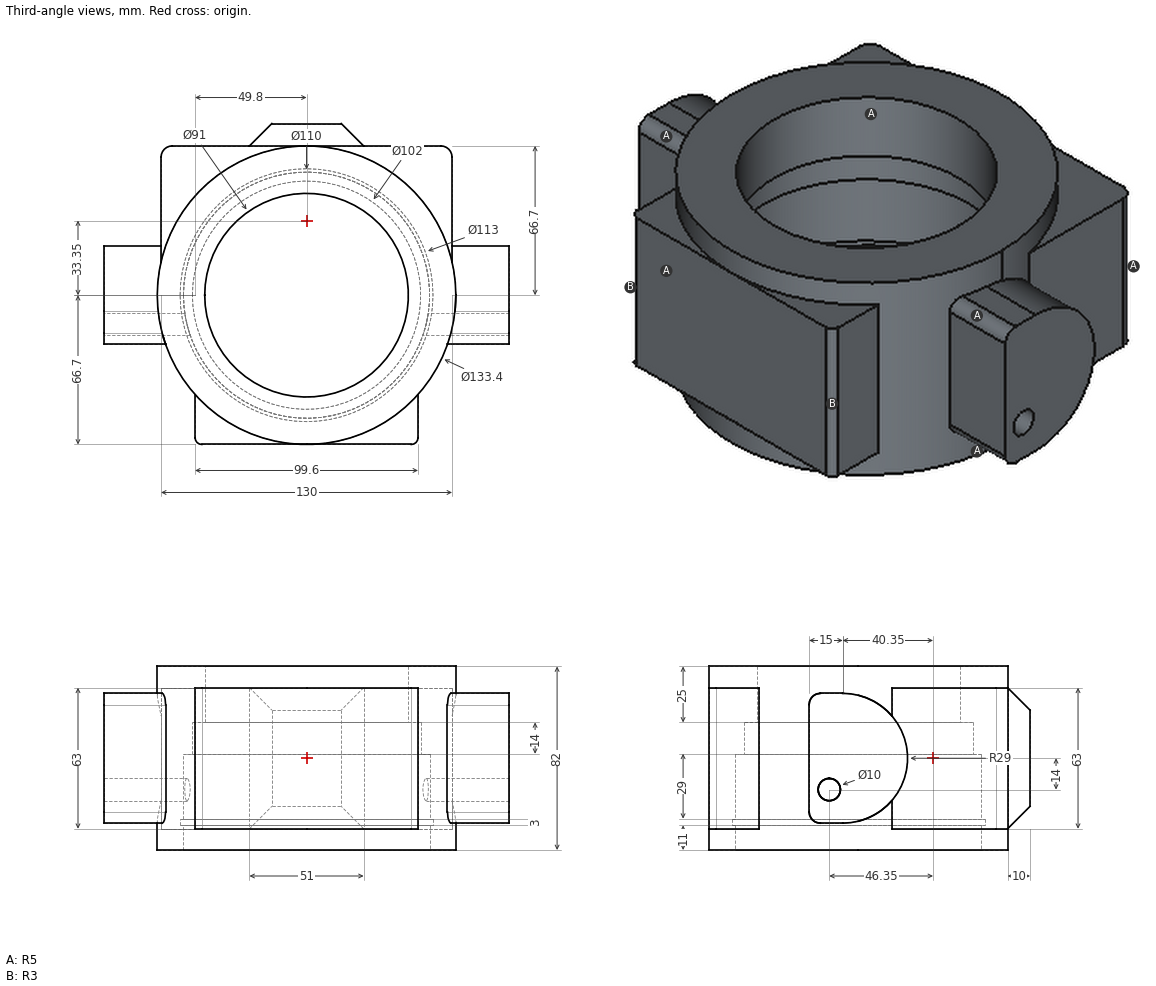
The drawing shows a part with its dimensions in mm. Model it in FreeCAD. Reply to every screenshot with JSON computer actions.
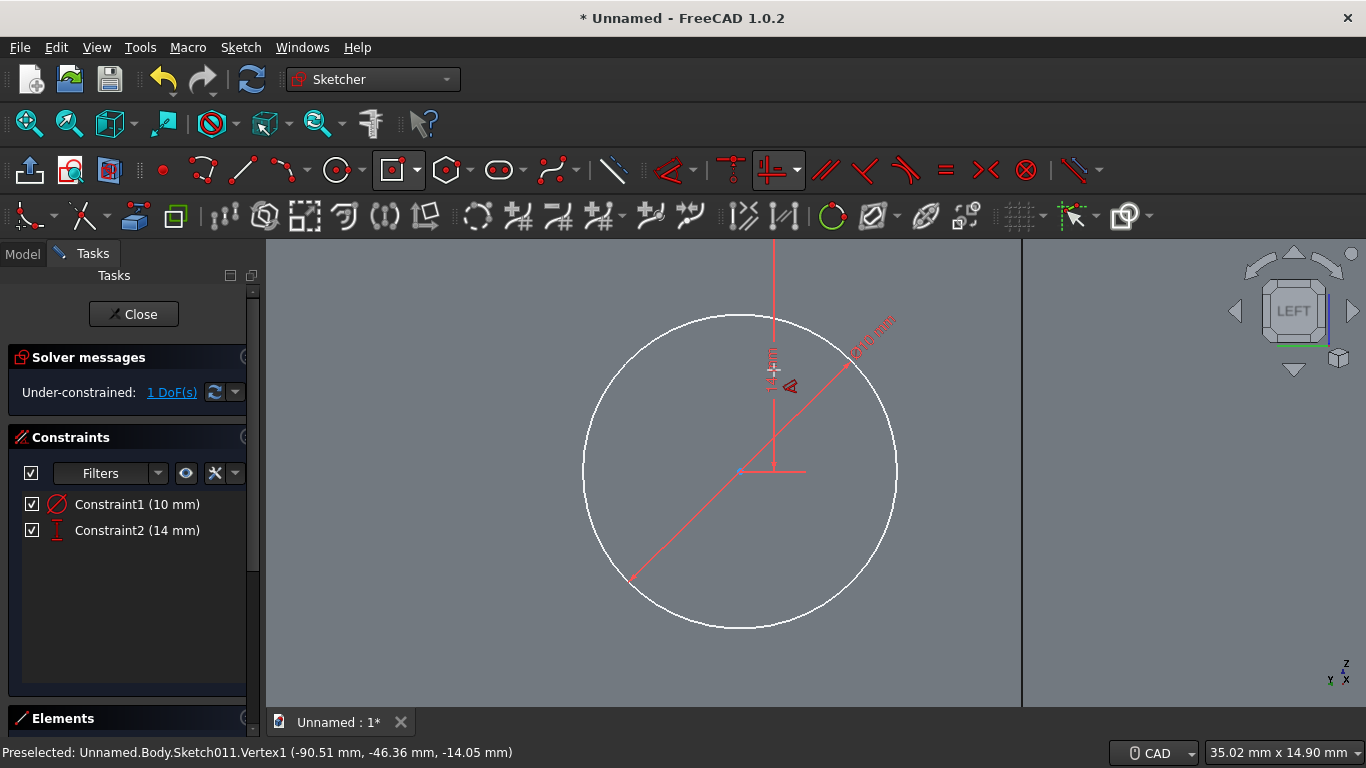
{"action": "left_click", "coordinate": [740, 472]}
{"action": "left_click", "coordinate": [517, 506]}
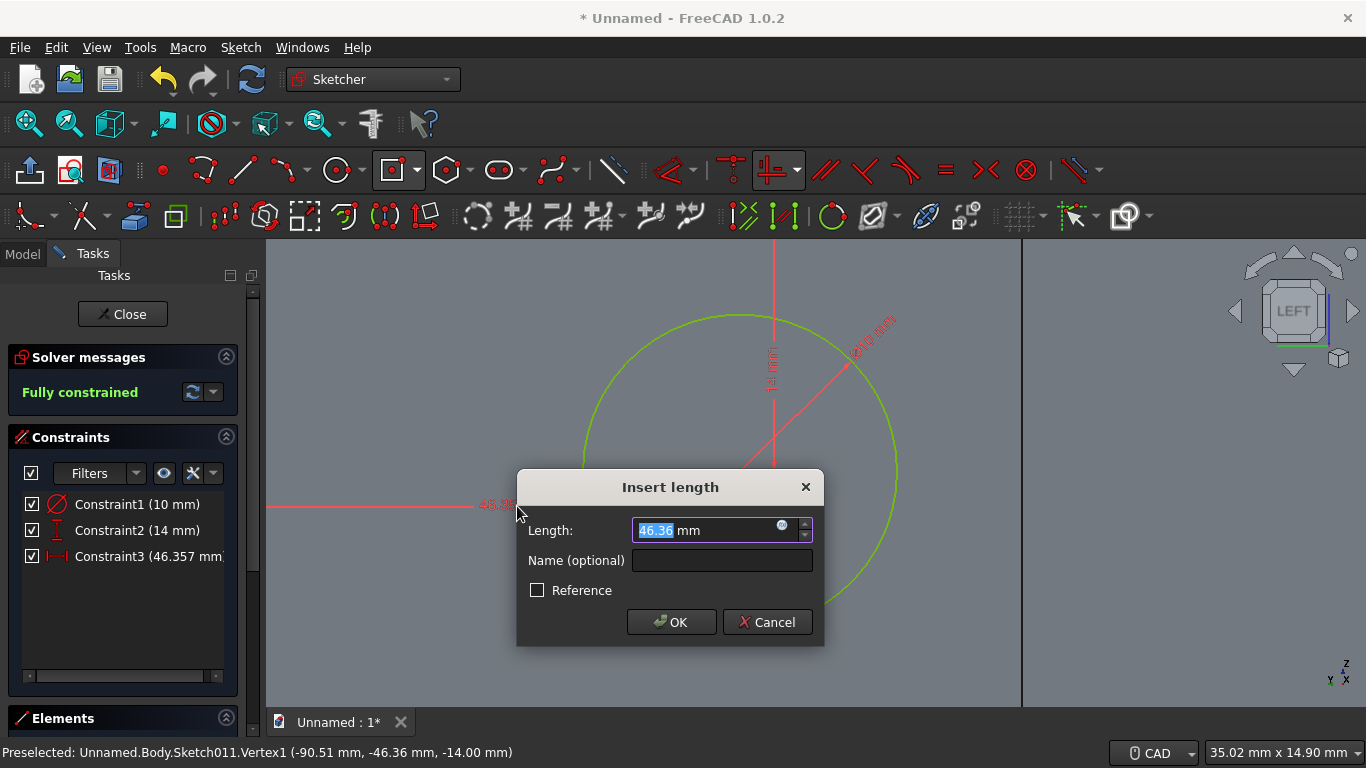
{"action": "type", "text": "46.35"}
{"action": "key", "text": "Return"}
{"action": "key", "text": "Escape"}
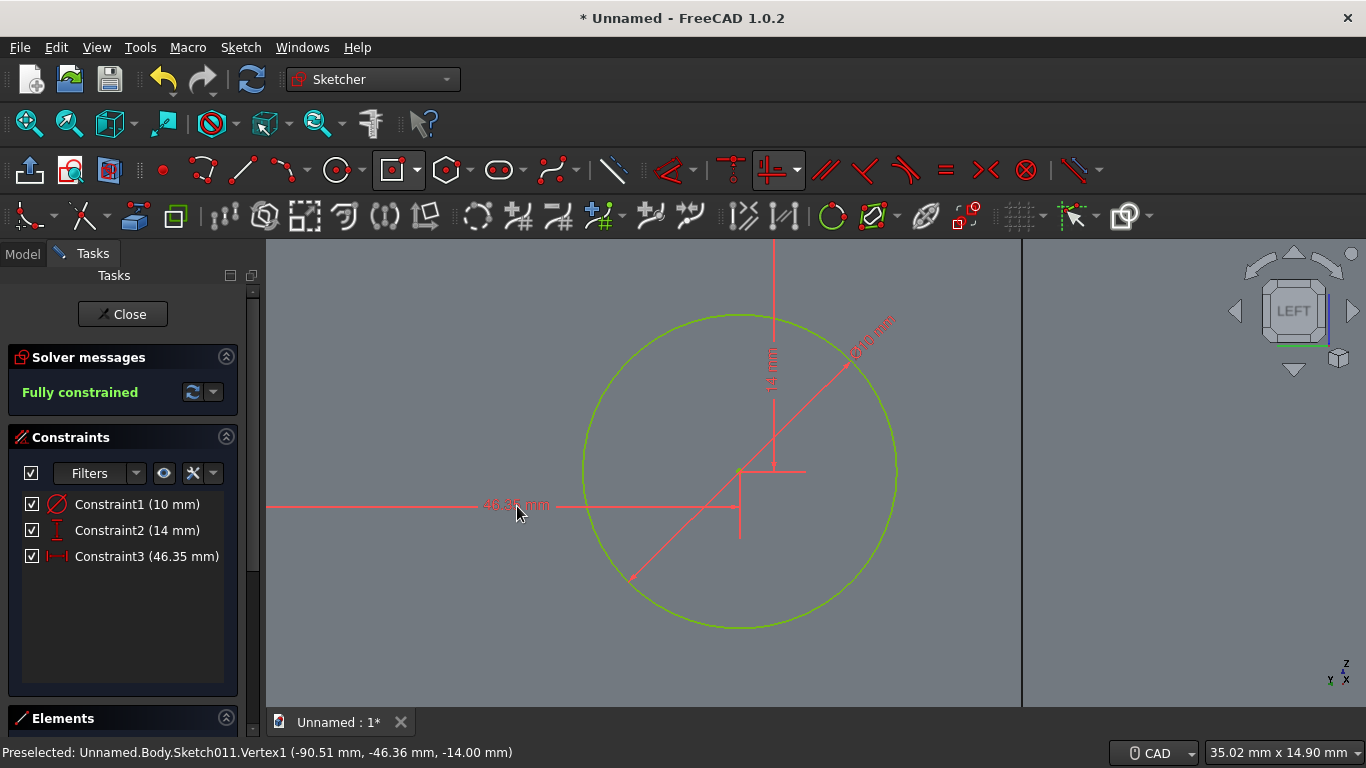
{"action": "left_click", "coordinate": [123, 314]}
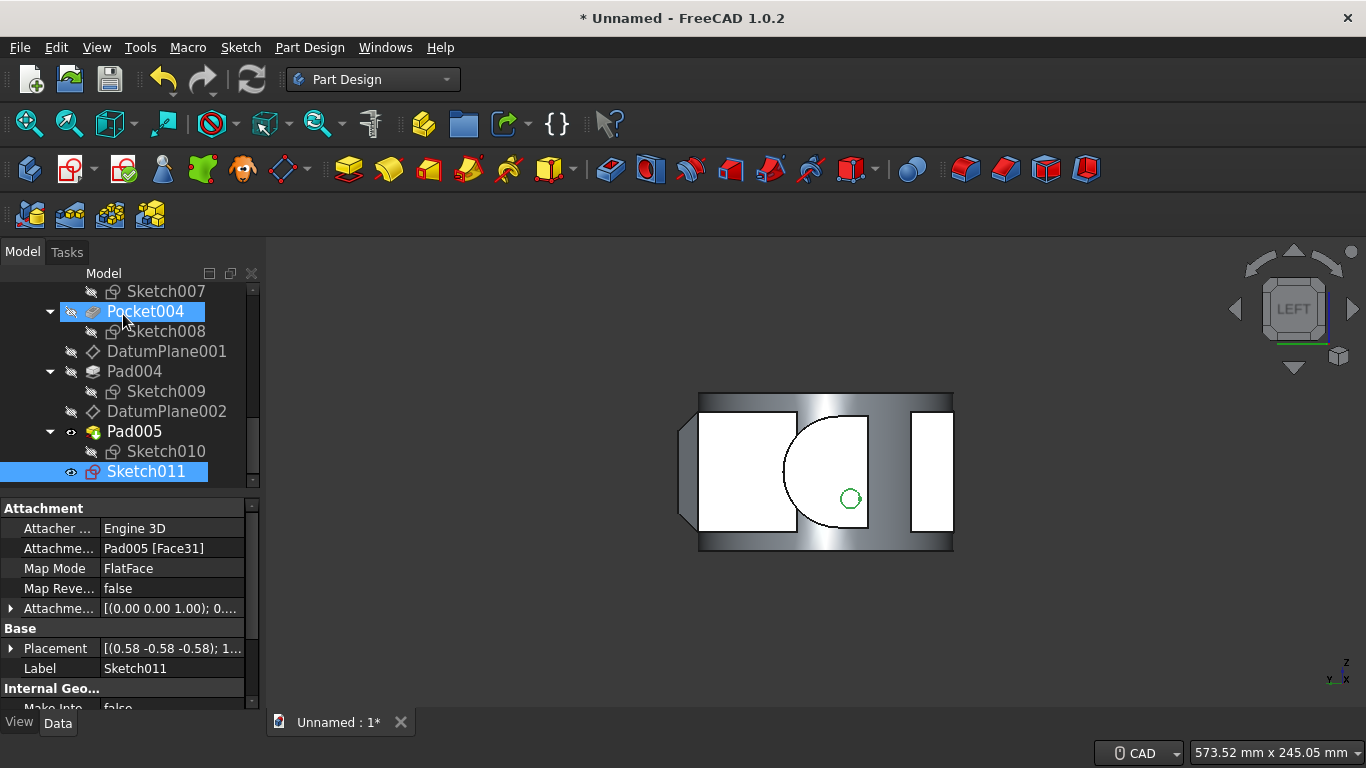
{"action": "left_click", "coordinate": [612, 170]}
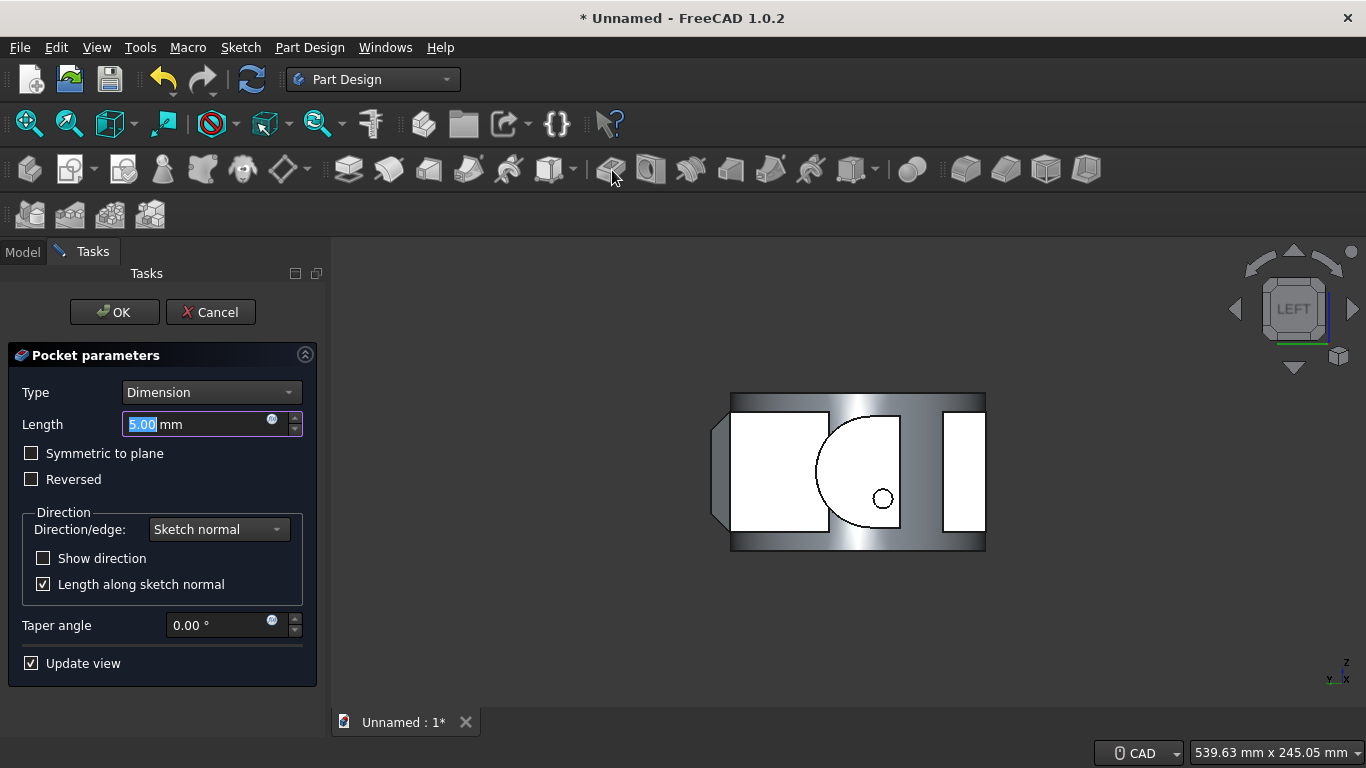
{"action": "left_click", "coordinate": [212, 392]}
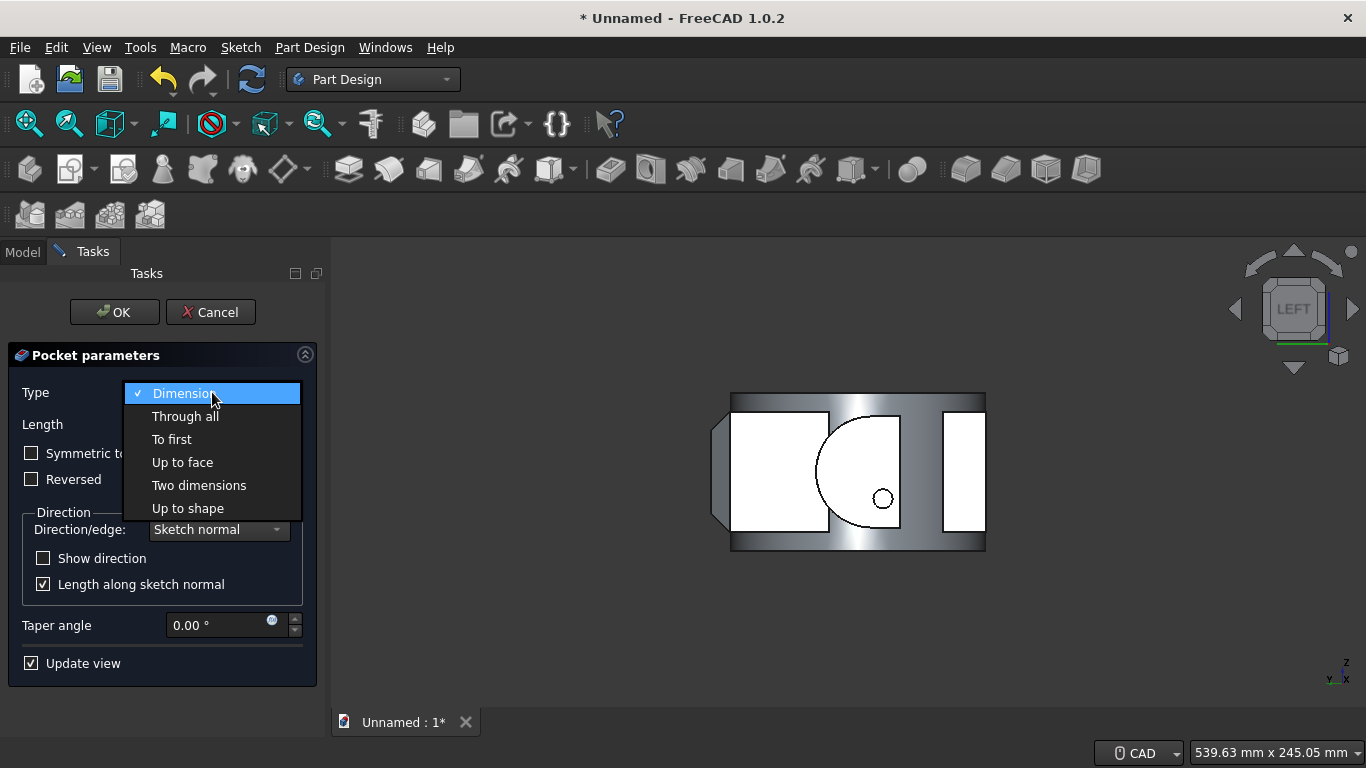
{"action": "left_click", "coordinate": [212, 416]}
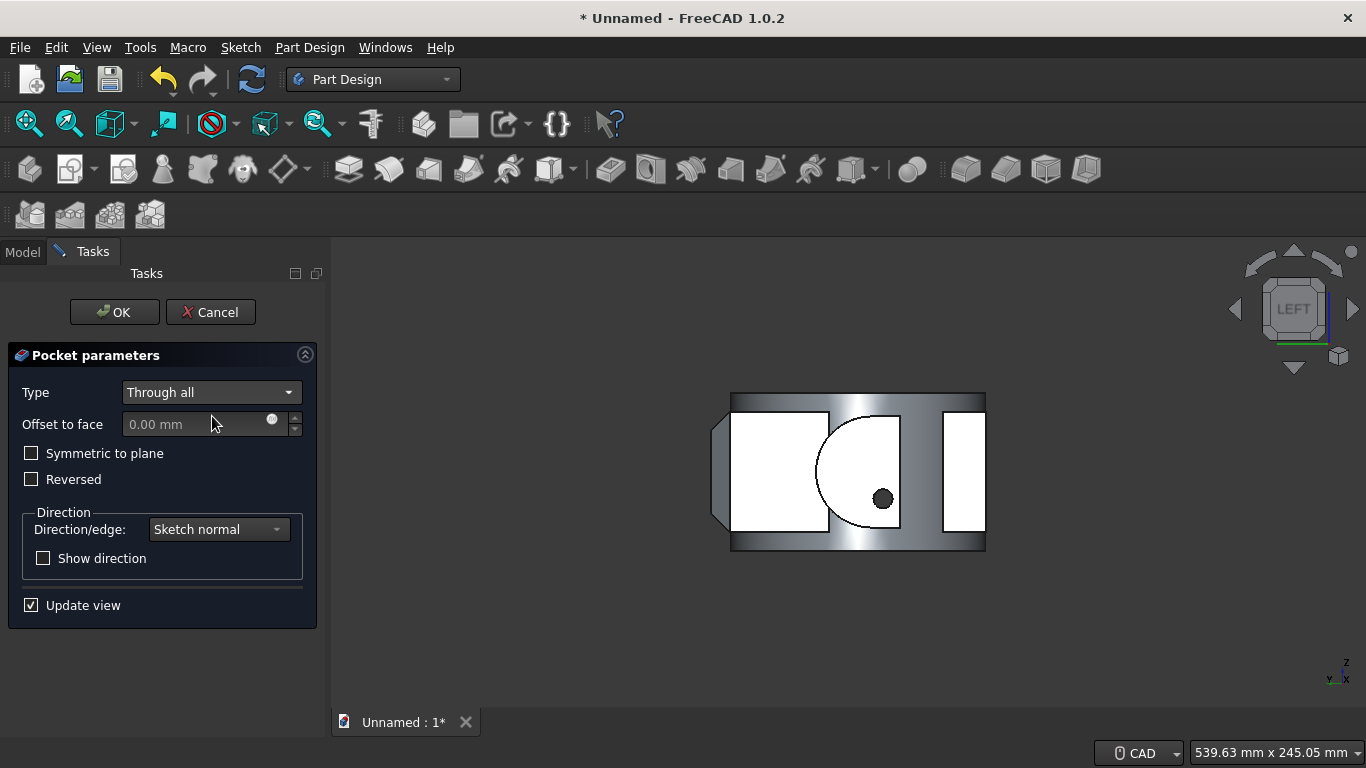
{"action": "left_click", "coordinate": [115, 312]}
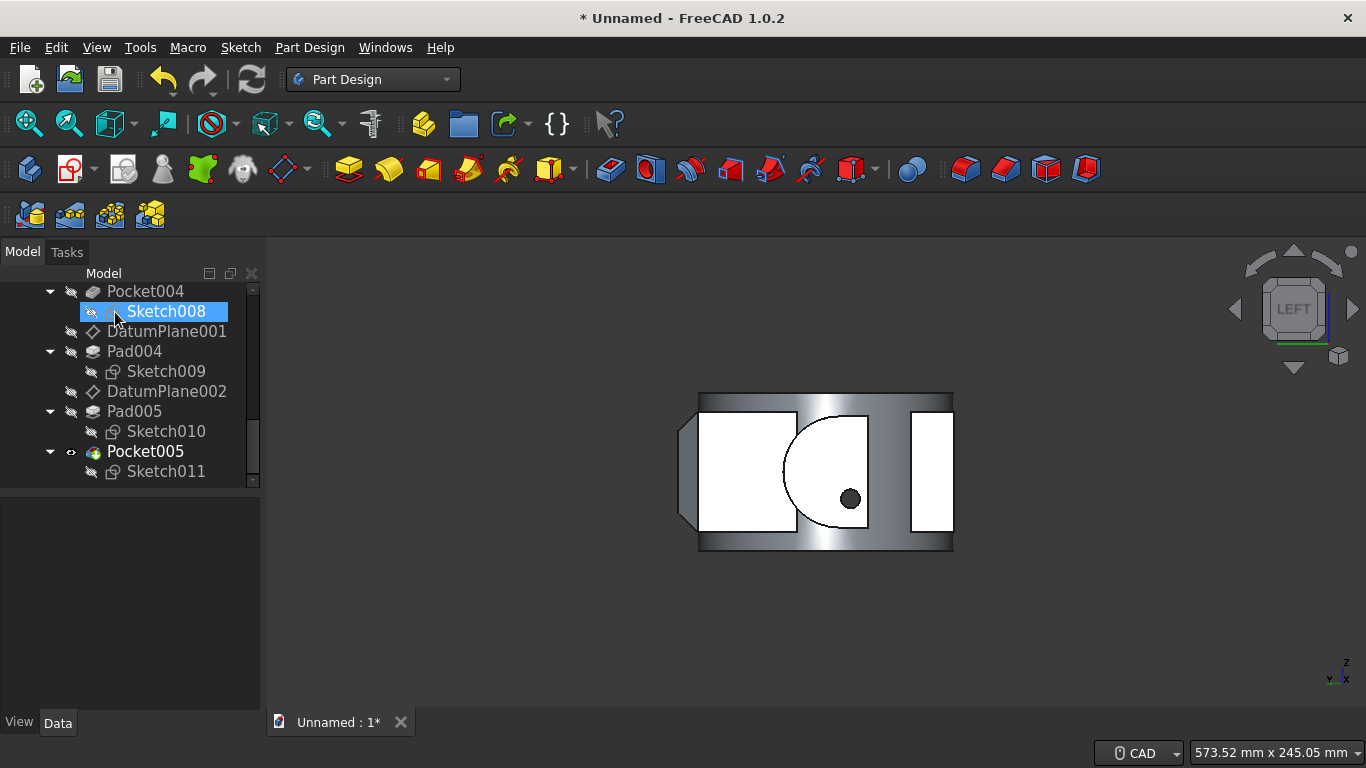
{"action": "left_click", "coordinate": [30, 124]}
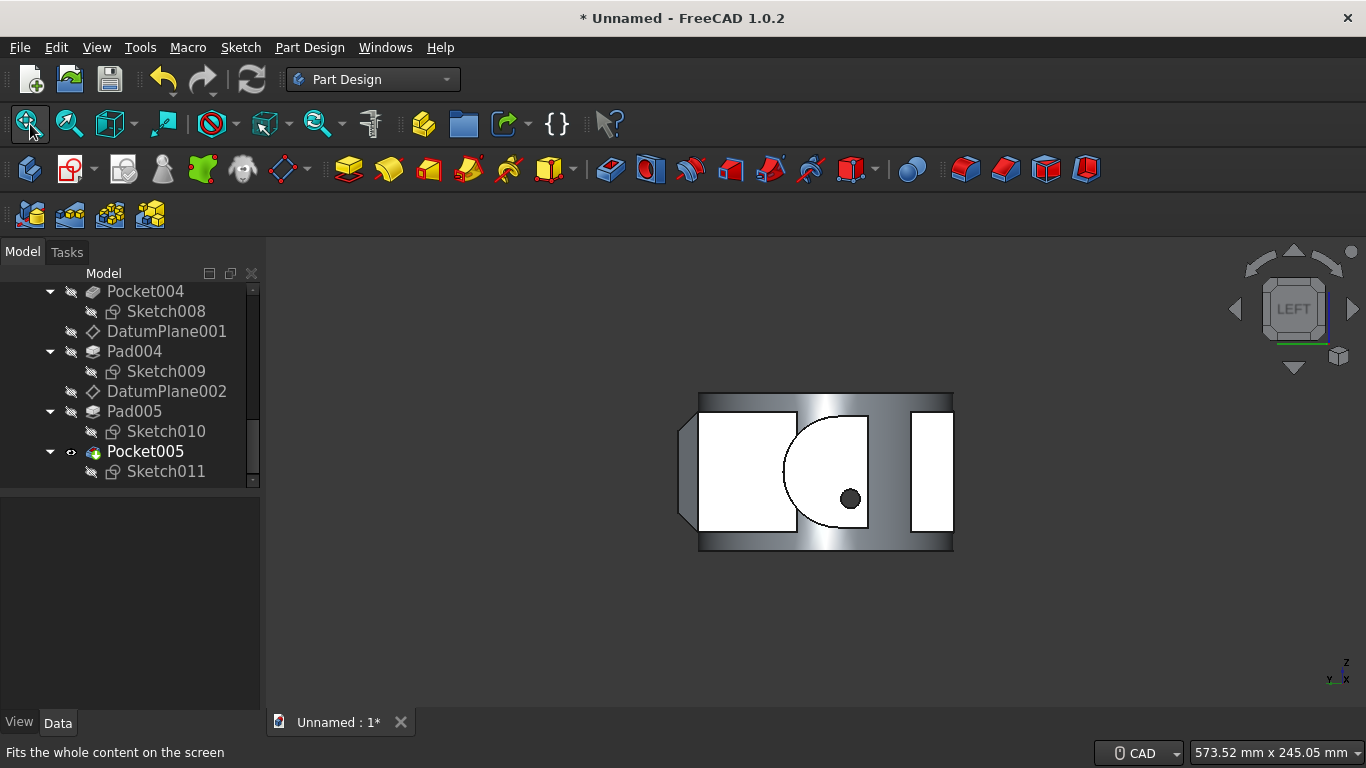
{"action": "left_click", "coordinate": [698, 471]}